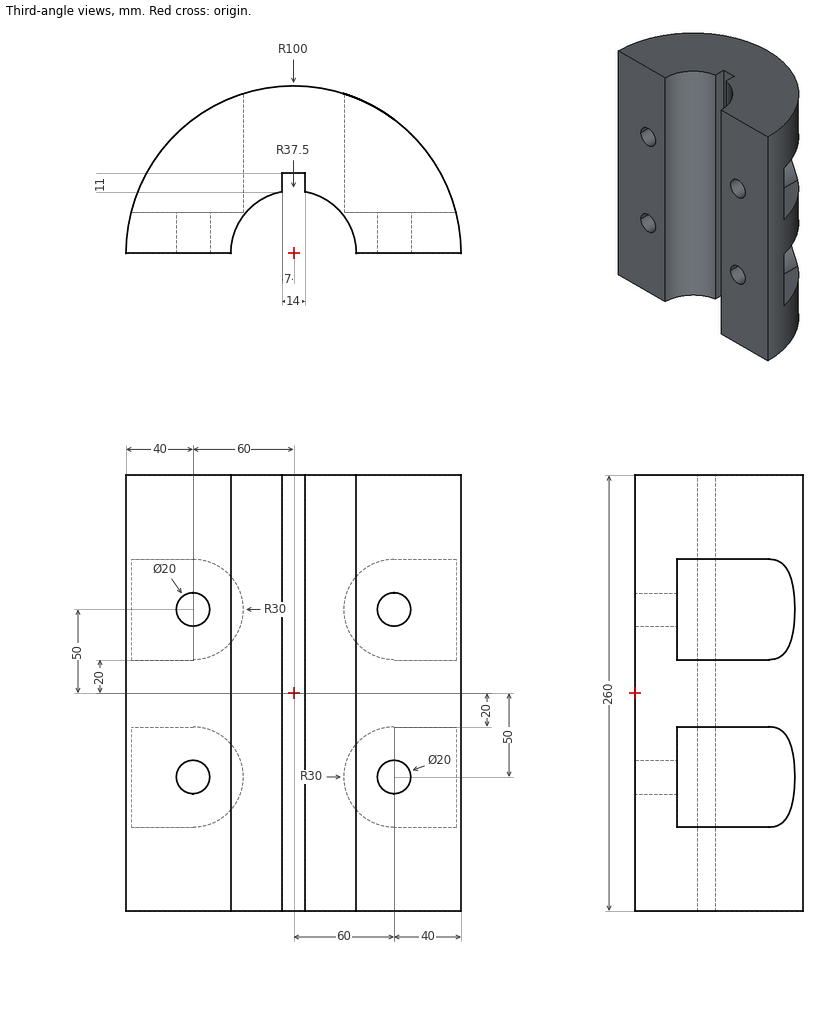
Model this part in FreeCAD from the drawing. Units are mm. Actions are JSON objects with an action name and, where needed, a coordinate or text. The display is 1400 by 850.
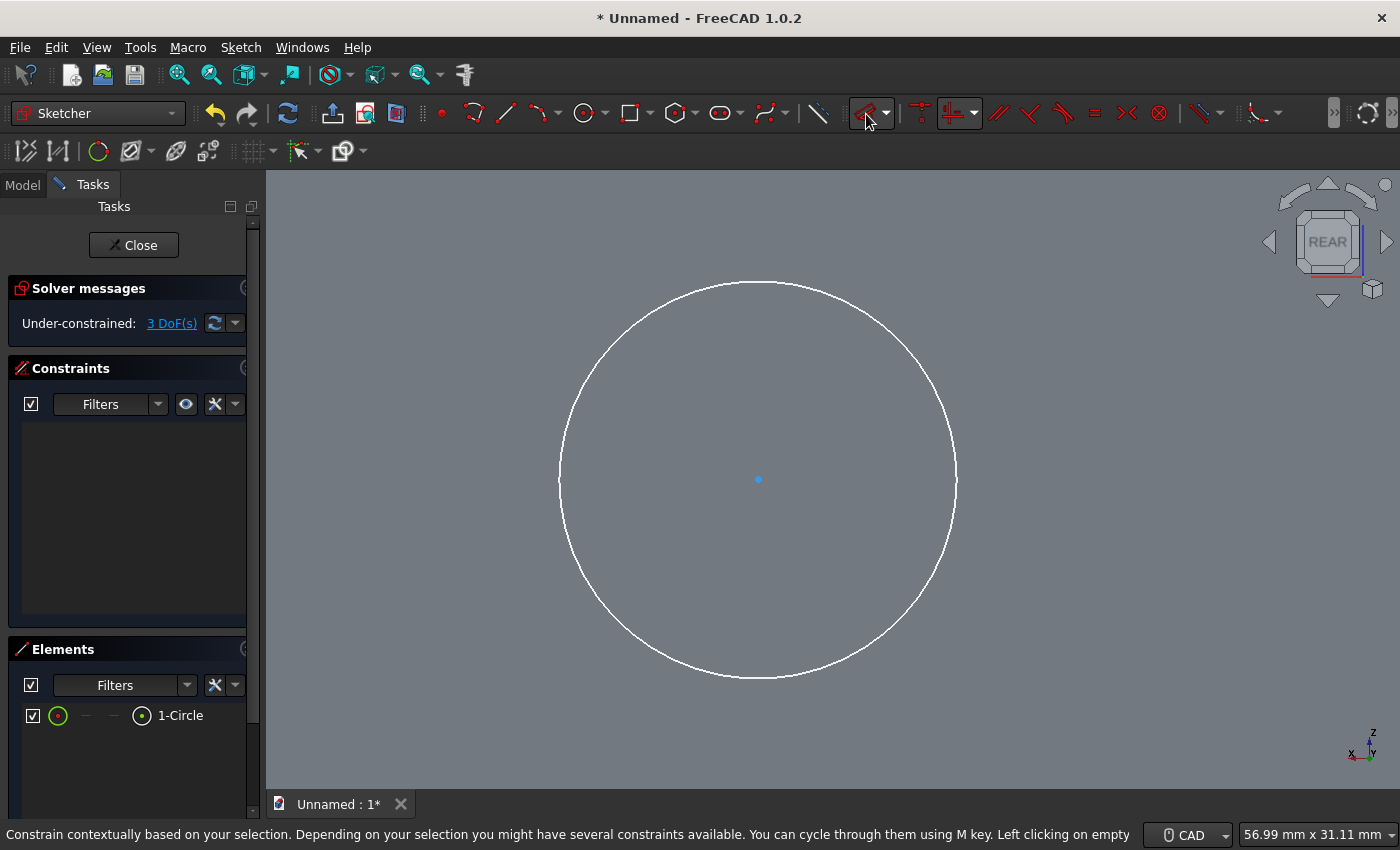
{"action": "left_click", "coordinate": [898, 339]}
{"action": "left_click", "coordinate": [921, 316]}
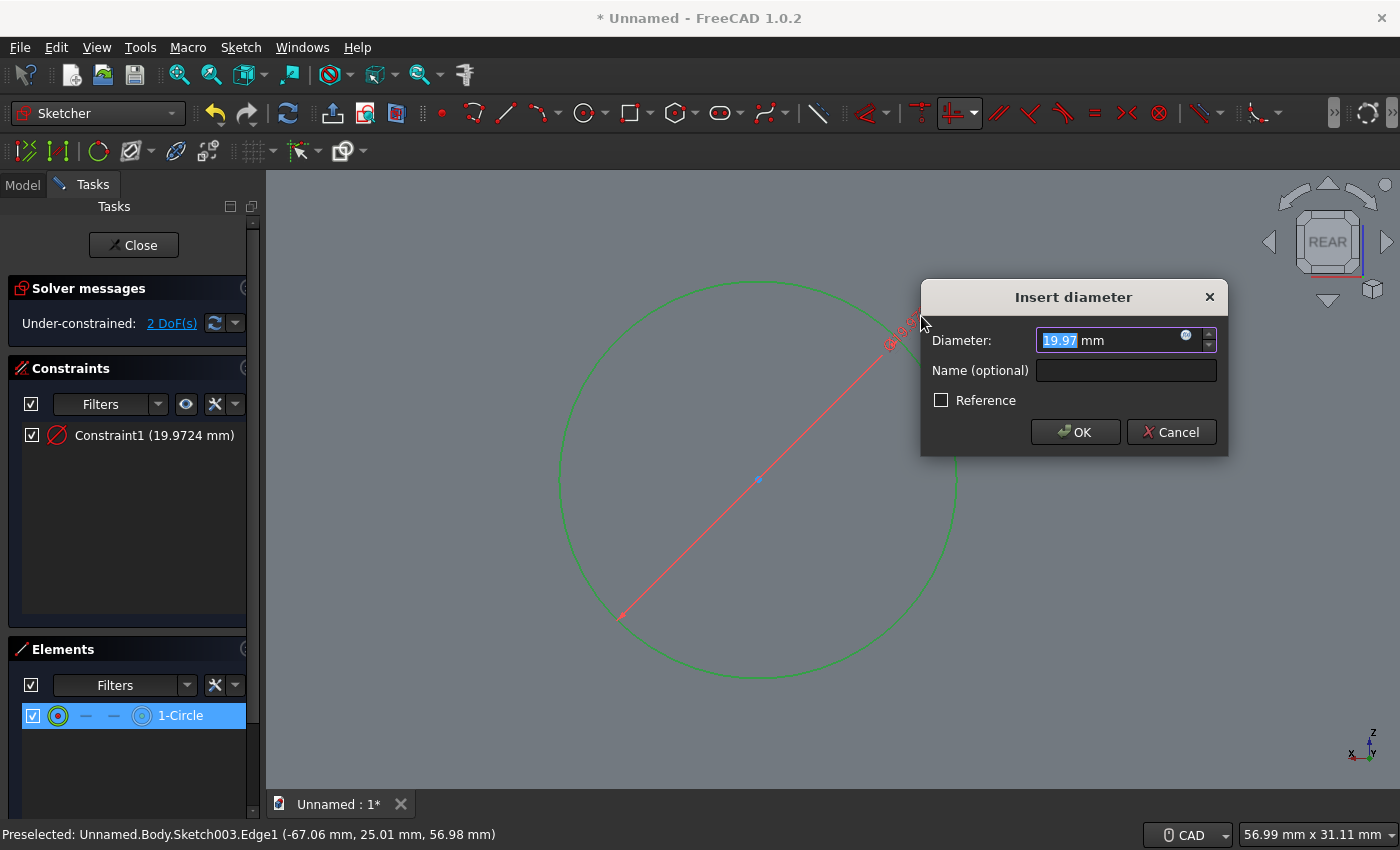
{"action": "type", "text": "20"}
{"action": "key", "text": "Return"}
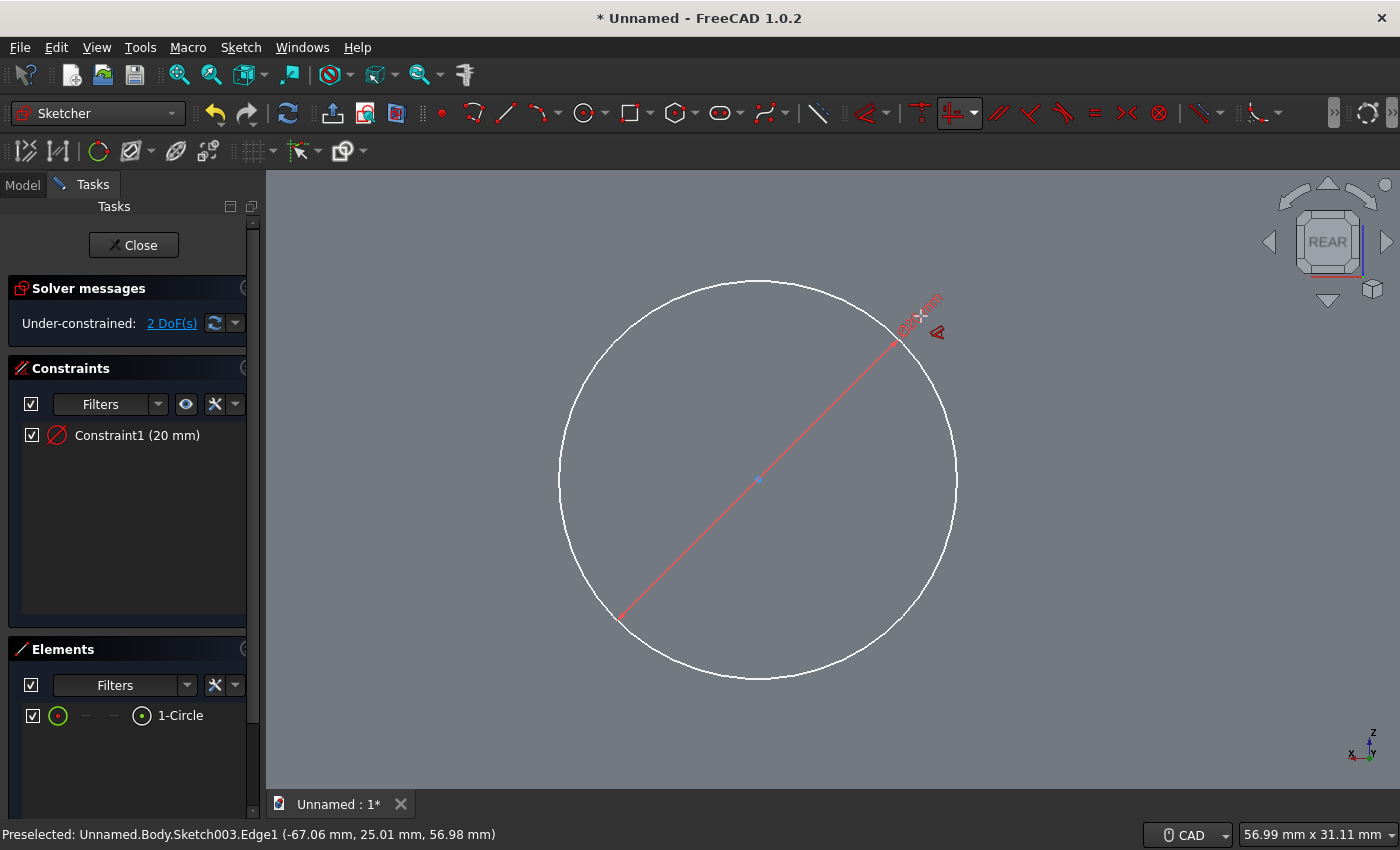
{"action": "left_click", "coordinate": [758, 480]}
{"action": "left_click", "coordinate": [526, 446]}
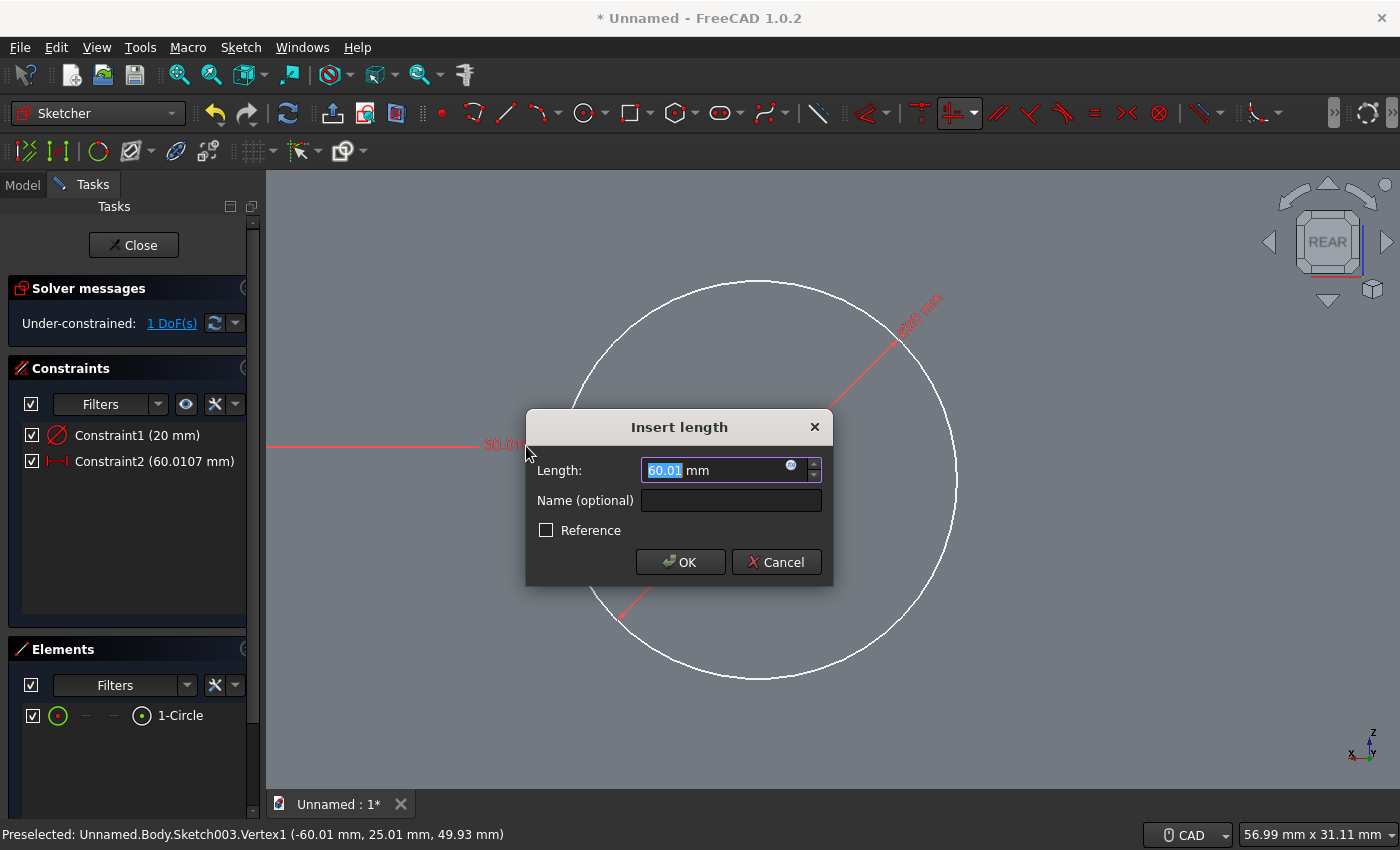
{"action": "type", "text": "60"}
{"action": "key", "text": "Return"}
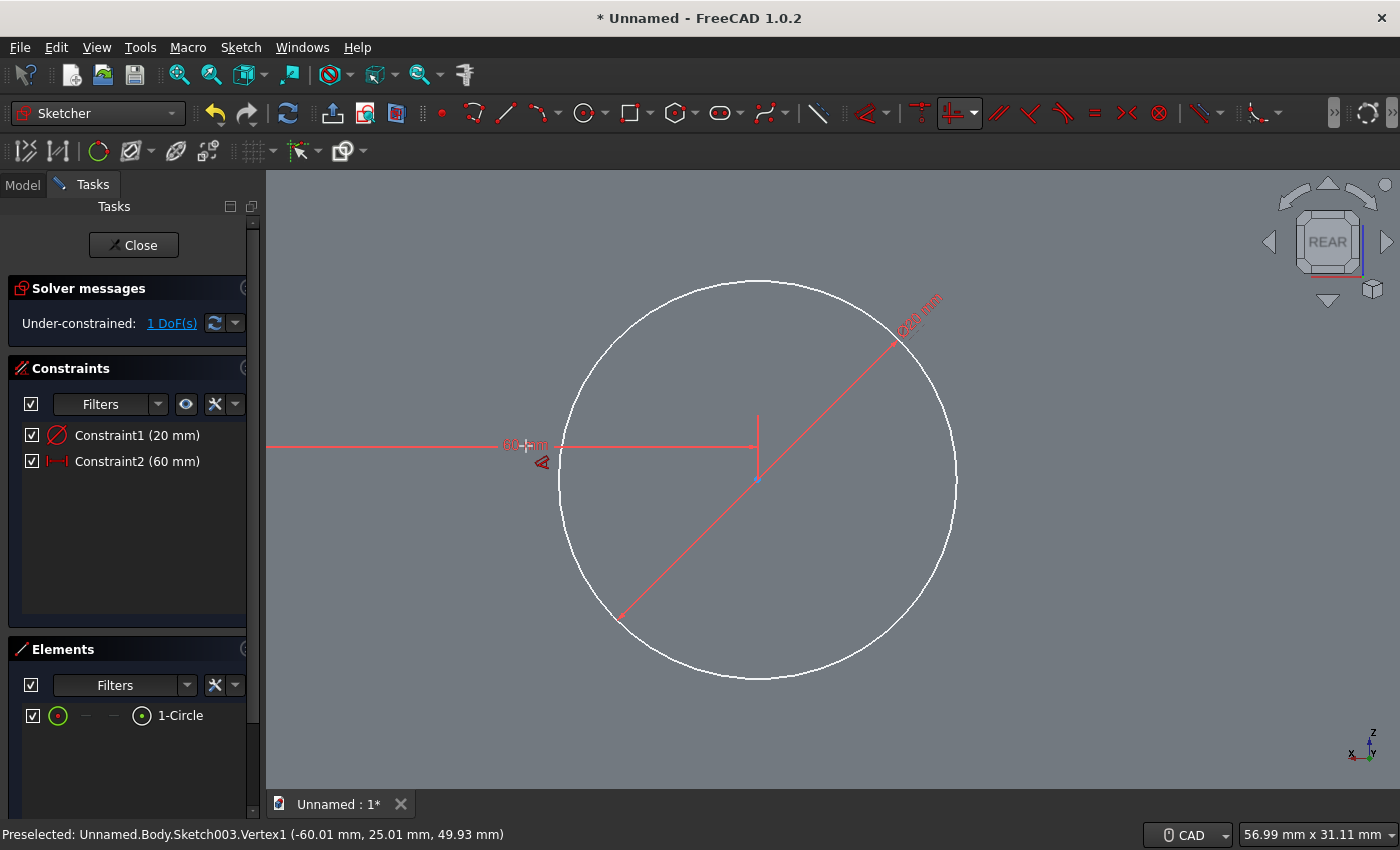
{"action": "left_click", "coordinate": [758, 480]}
{"action": "left_click", "coordinate": [792, 620]}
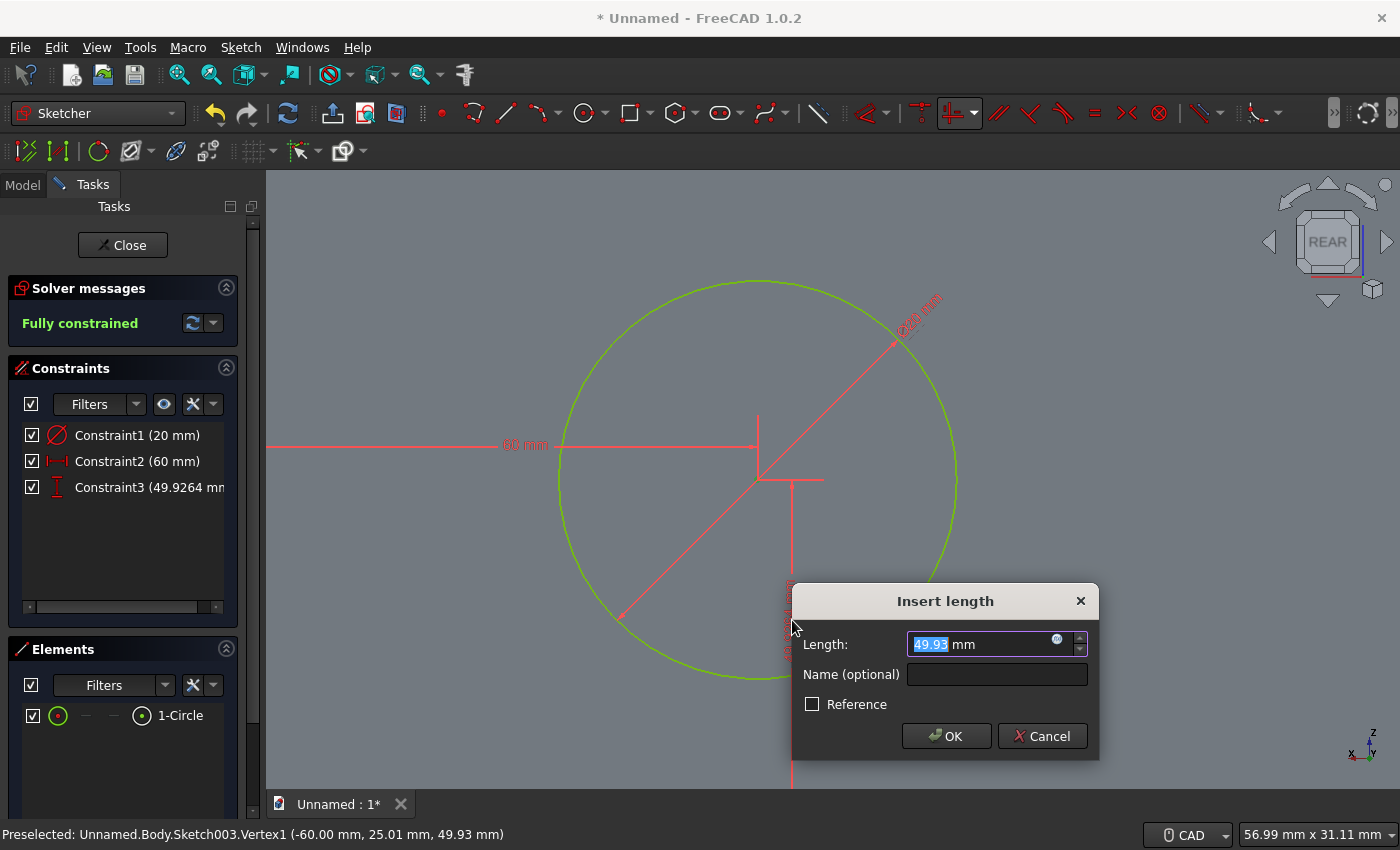
{"action": "type", "text": "50"}
{"action": "key", "text": "Return"}
{"action": "key", "text": "Escape"}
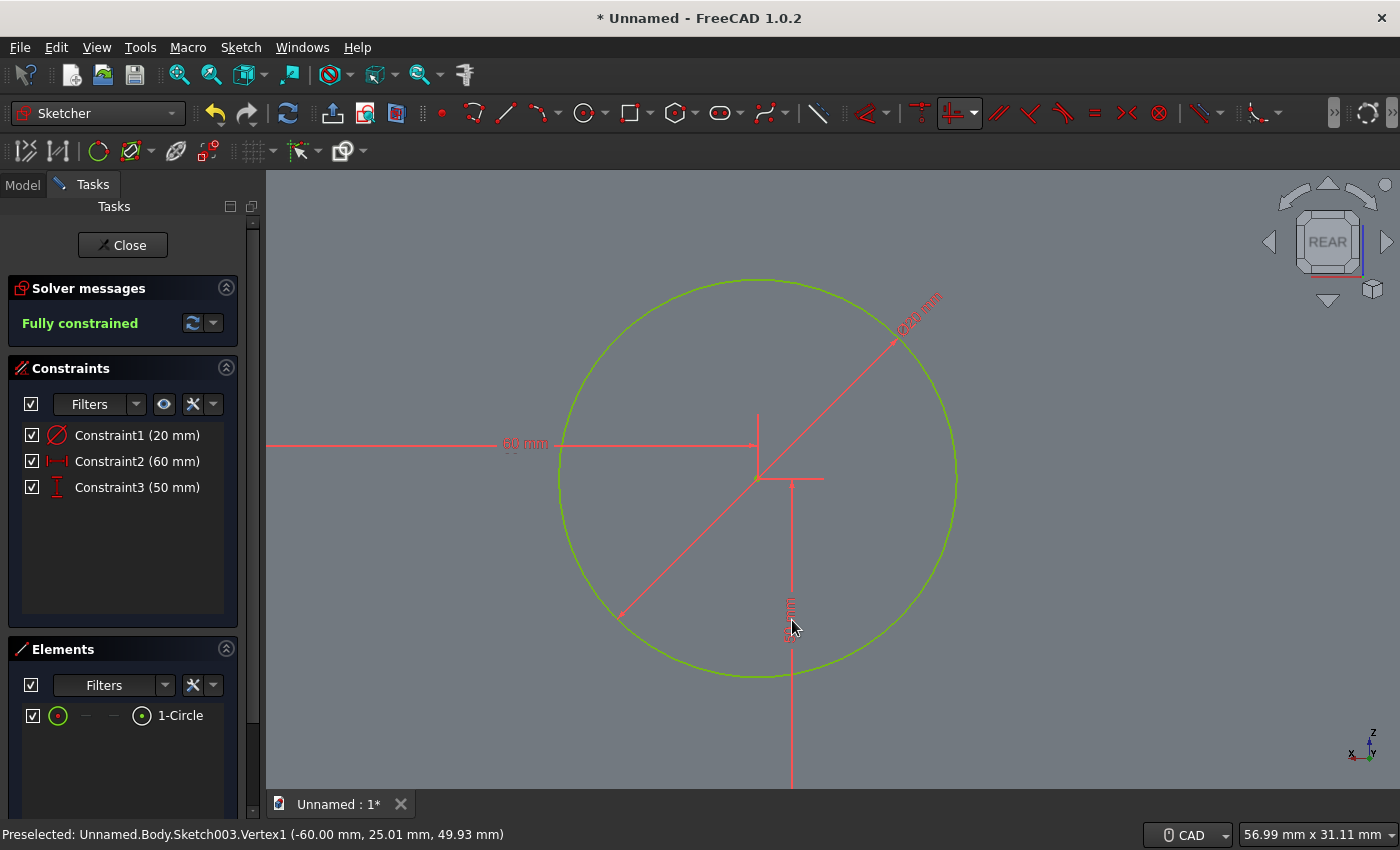
{"action": "left_click", "coordinate": [123, 245]}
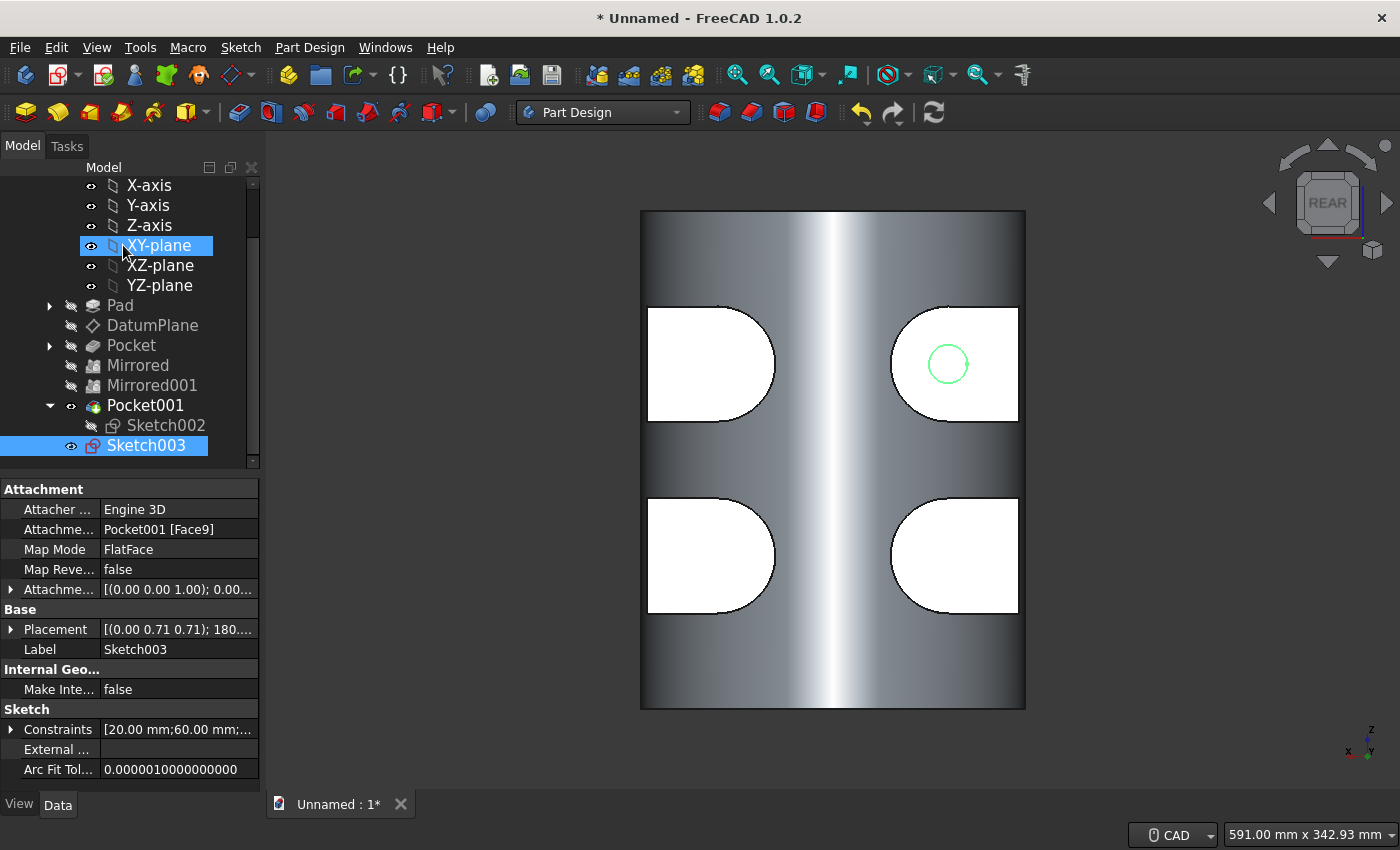
{"action": "left_click", "coordinate": [240, 112]}